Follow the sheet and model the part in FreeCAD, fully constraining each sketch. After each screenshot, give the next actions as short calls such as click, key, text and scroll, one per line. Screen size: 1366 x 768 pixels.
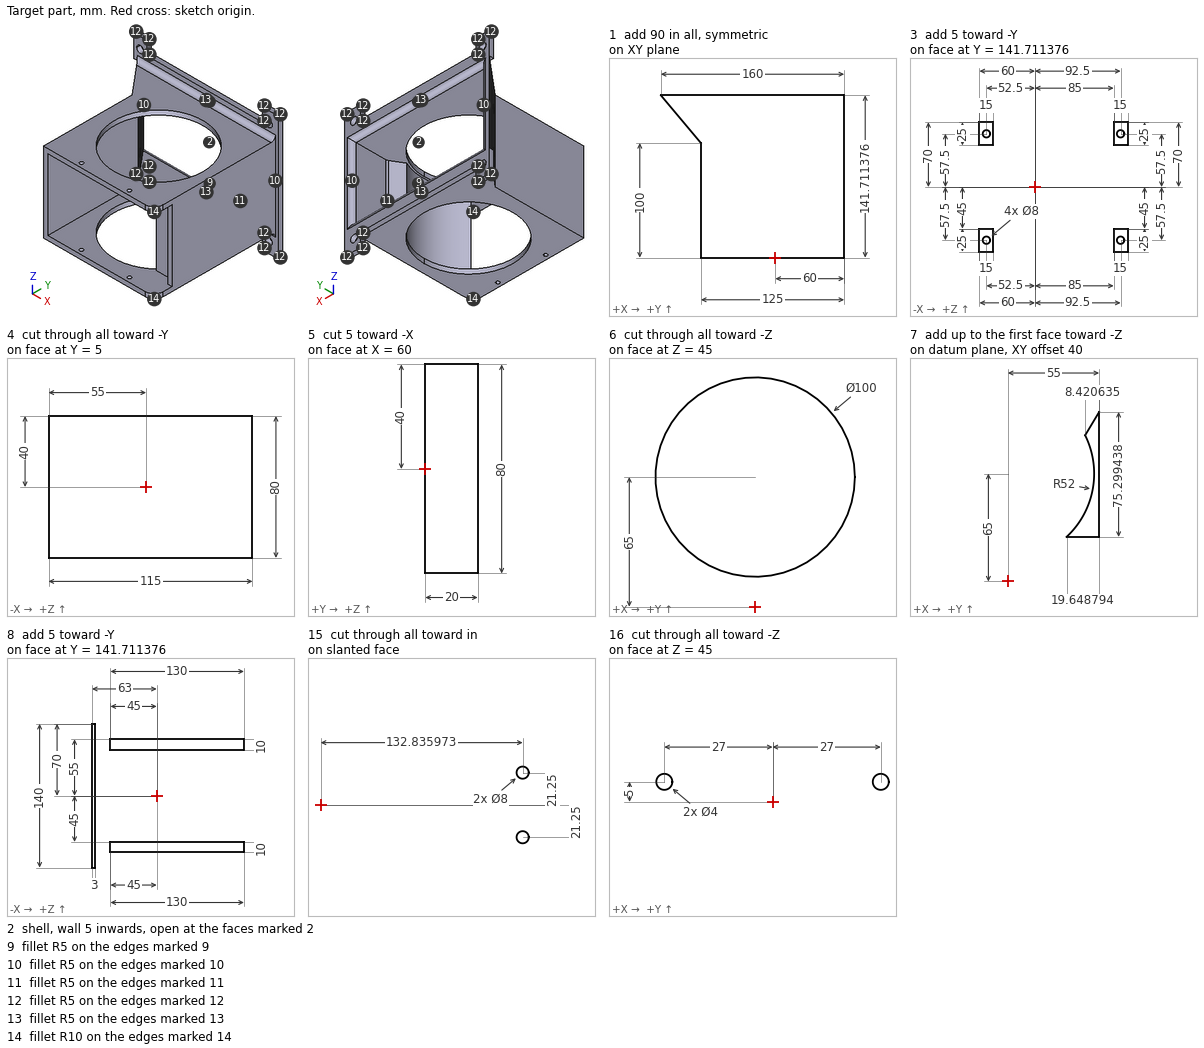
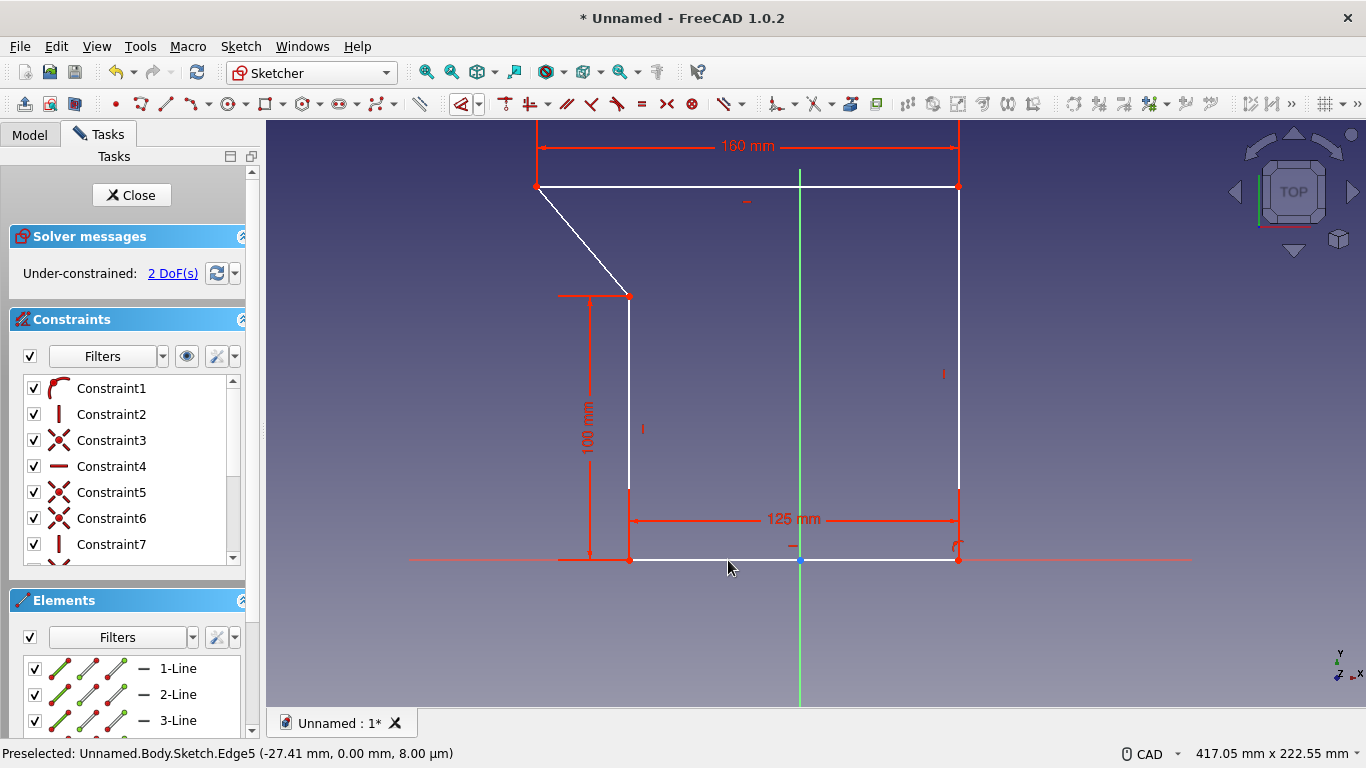
click(959, 560)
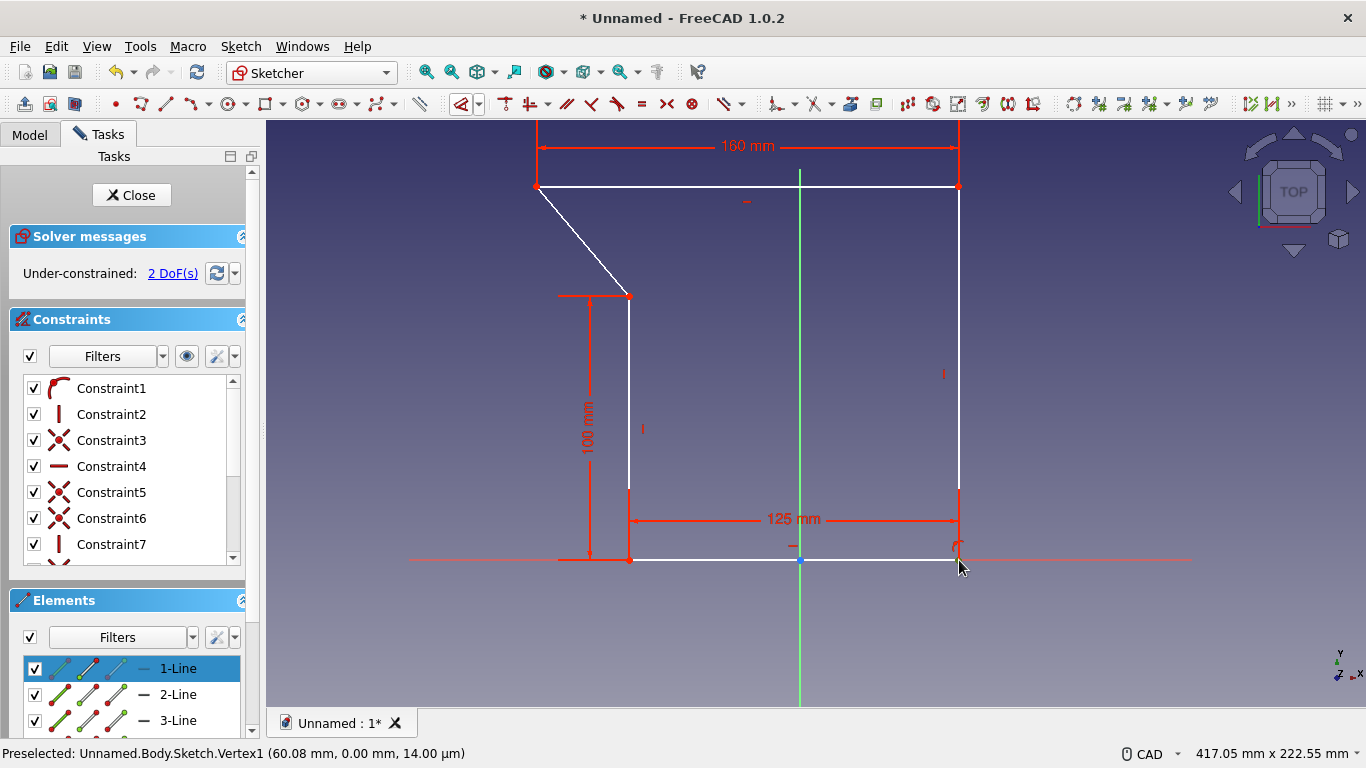
key(l)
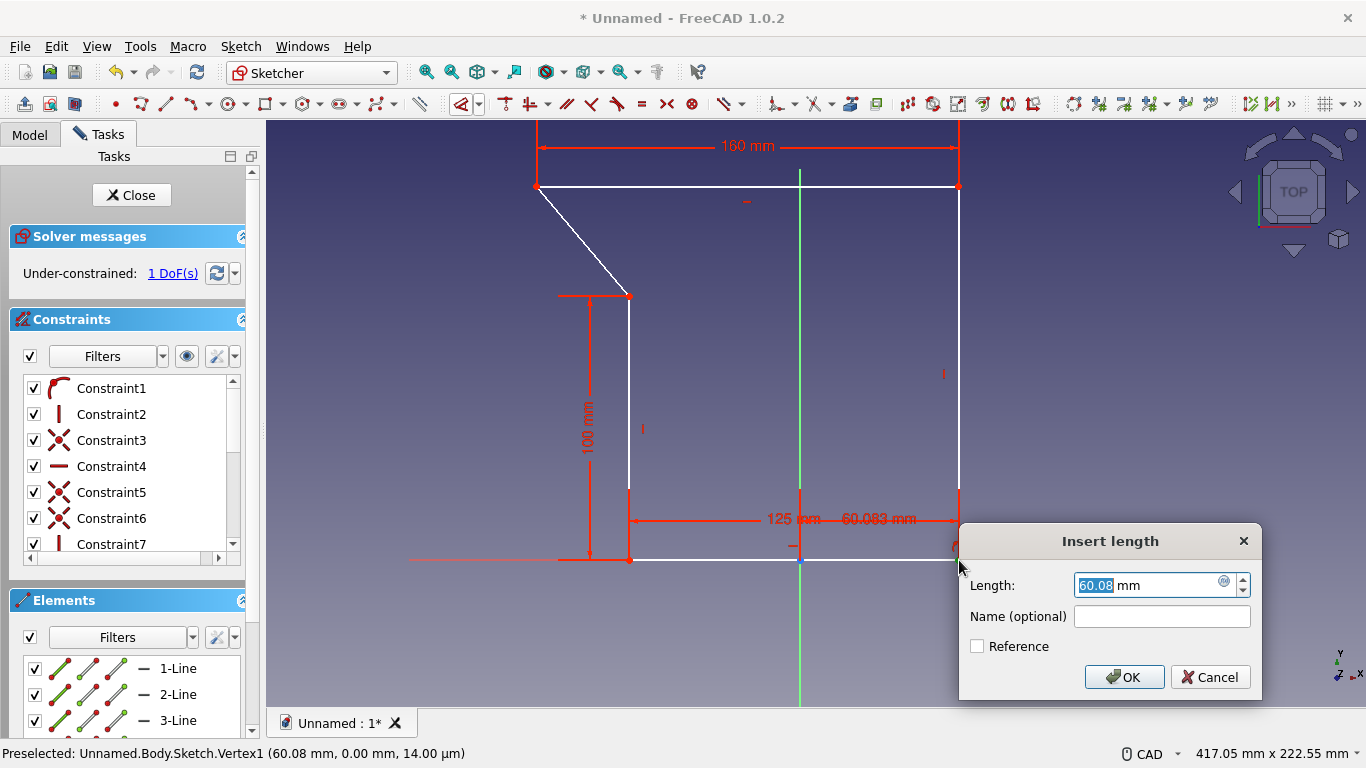
text(60)
key(Return)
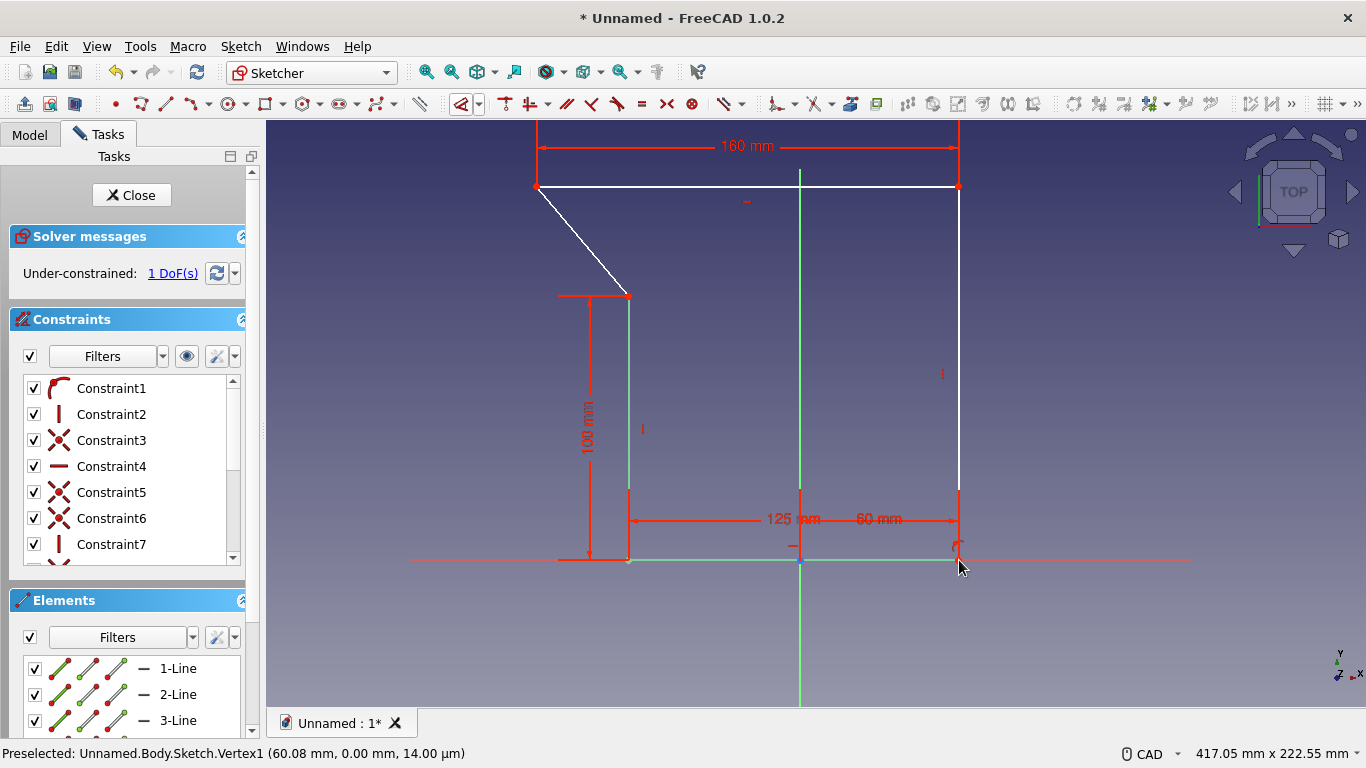
click(959, 448)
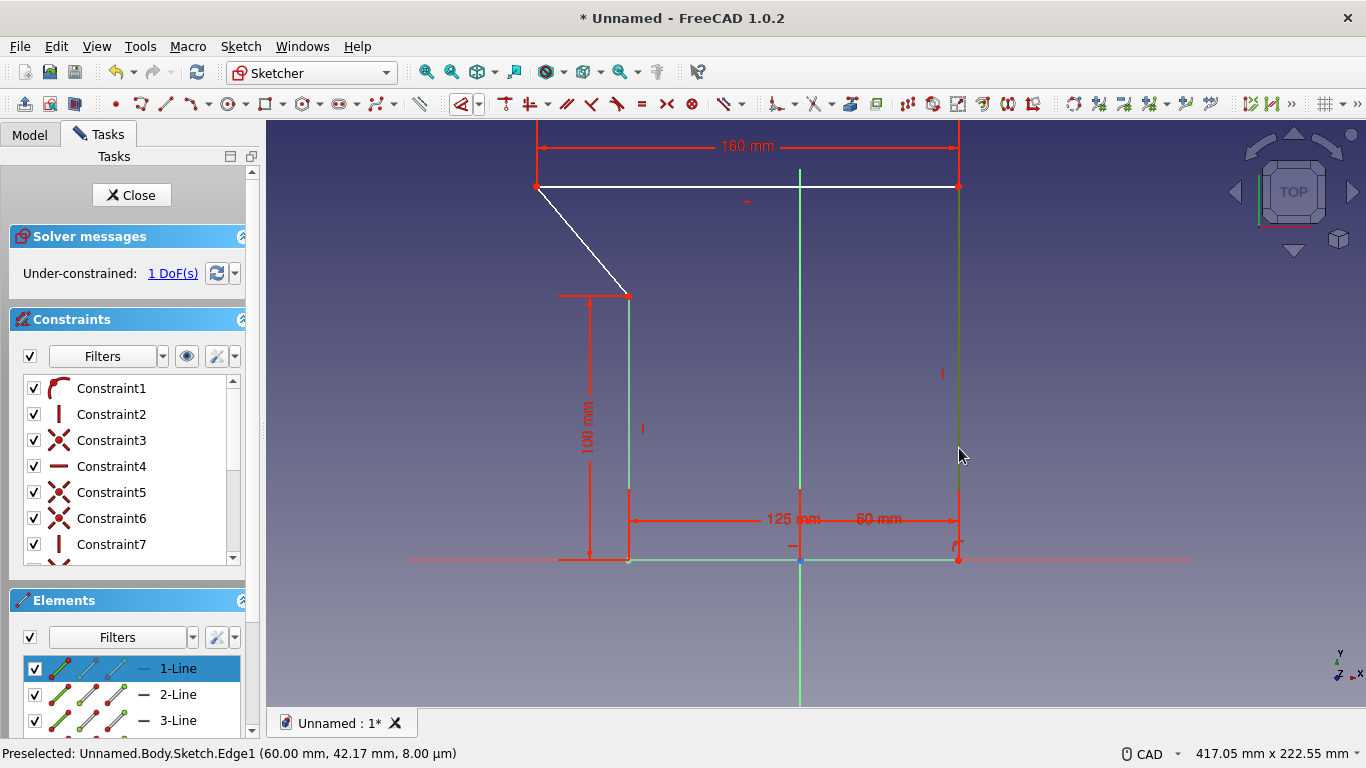
key(i)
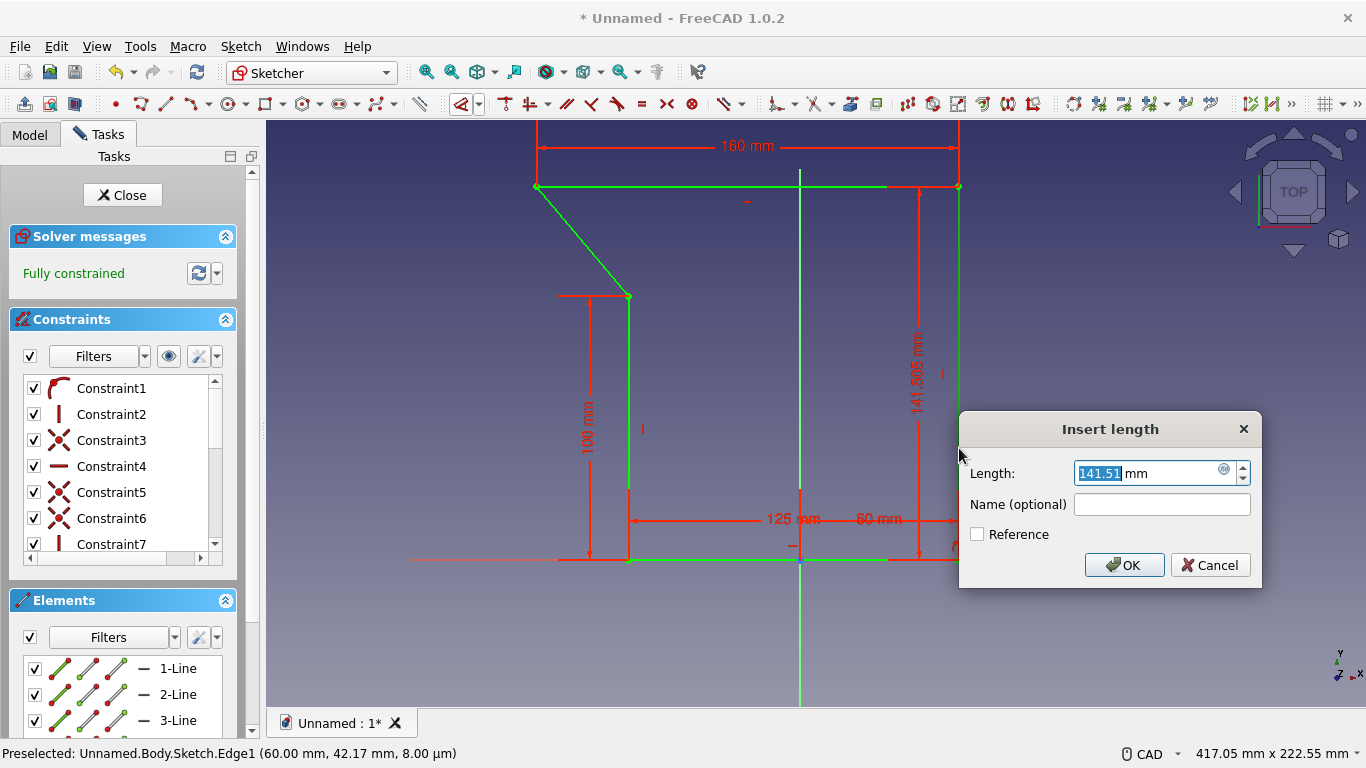
text(141.711376)
key(Return)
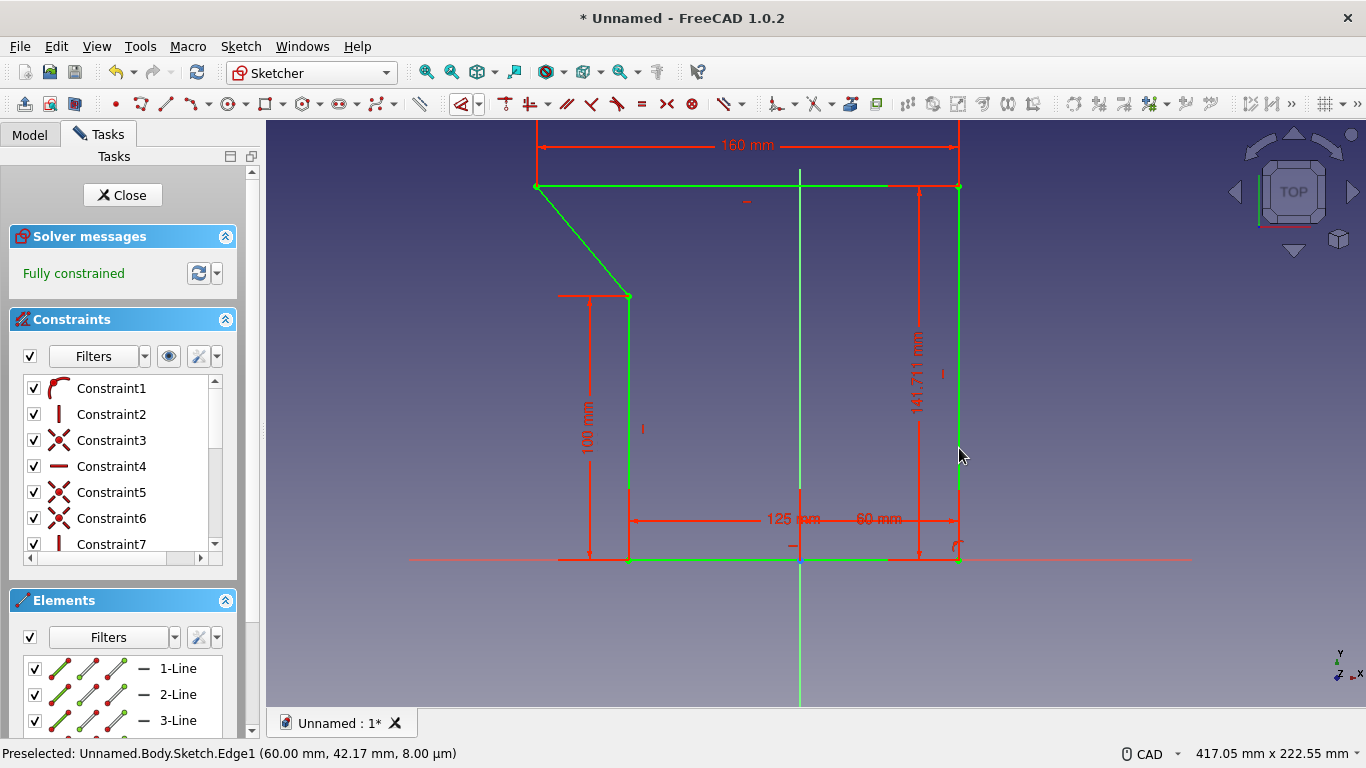
click(123, 195)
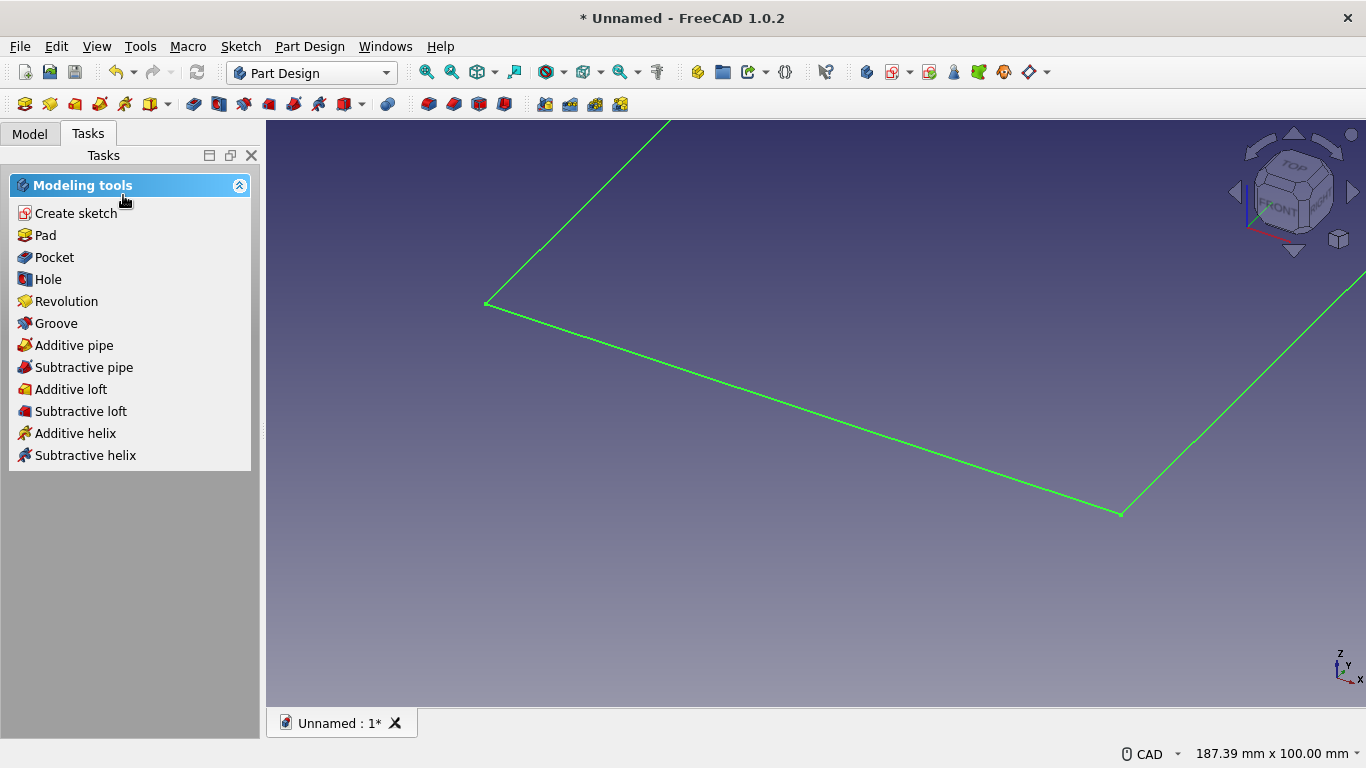
click(25, 104)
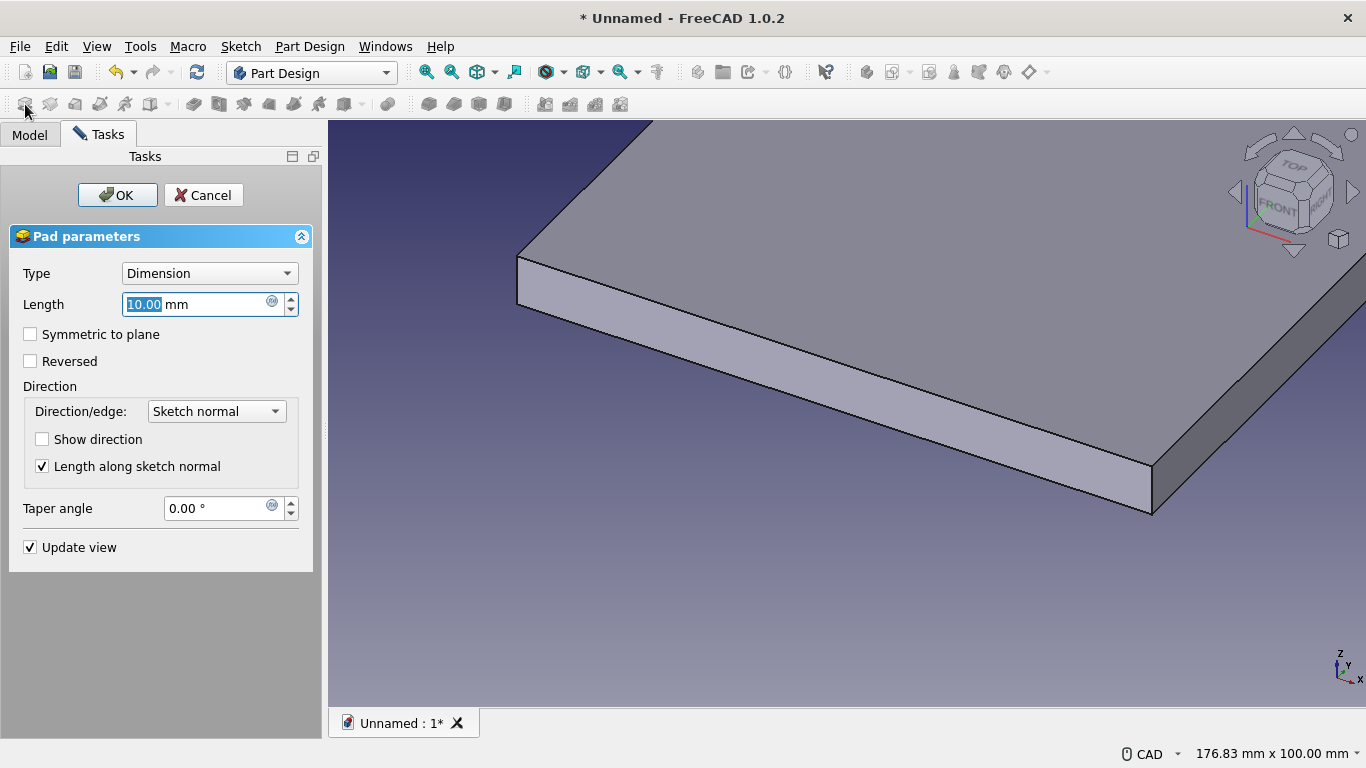
text(90)
key(Tab)